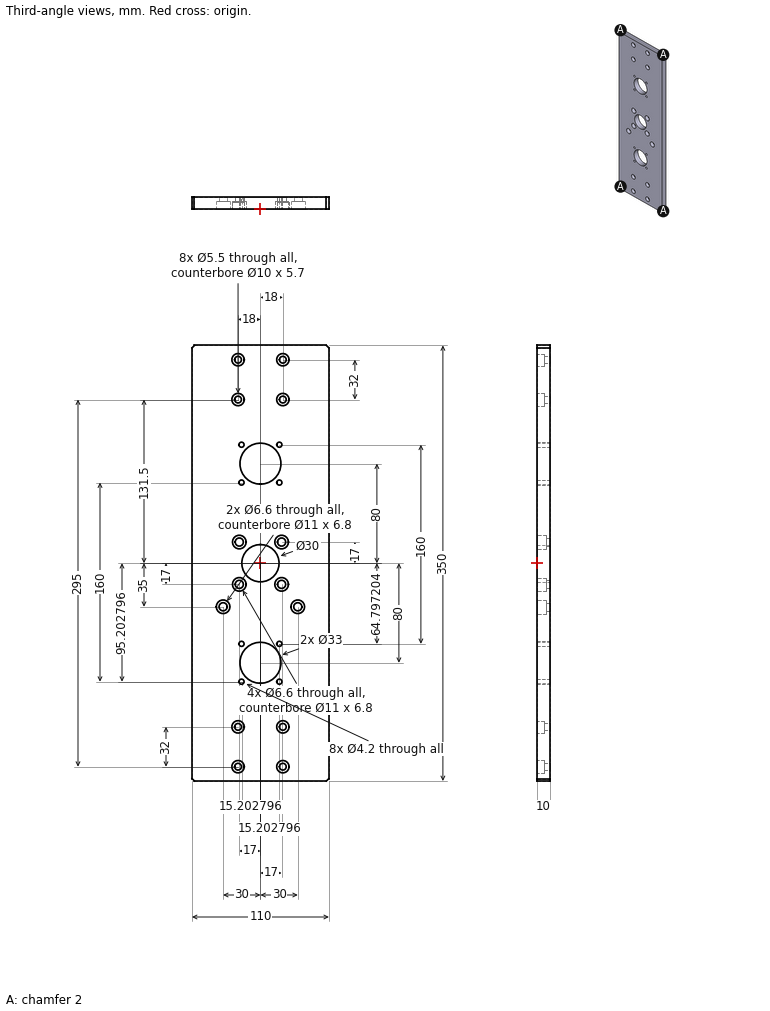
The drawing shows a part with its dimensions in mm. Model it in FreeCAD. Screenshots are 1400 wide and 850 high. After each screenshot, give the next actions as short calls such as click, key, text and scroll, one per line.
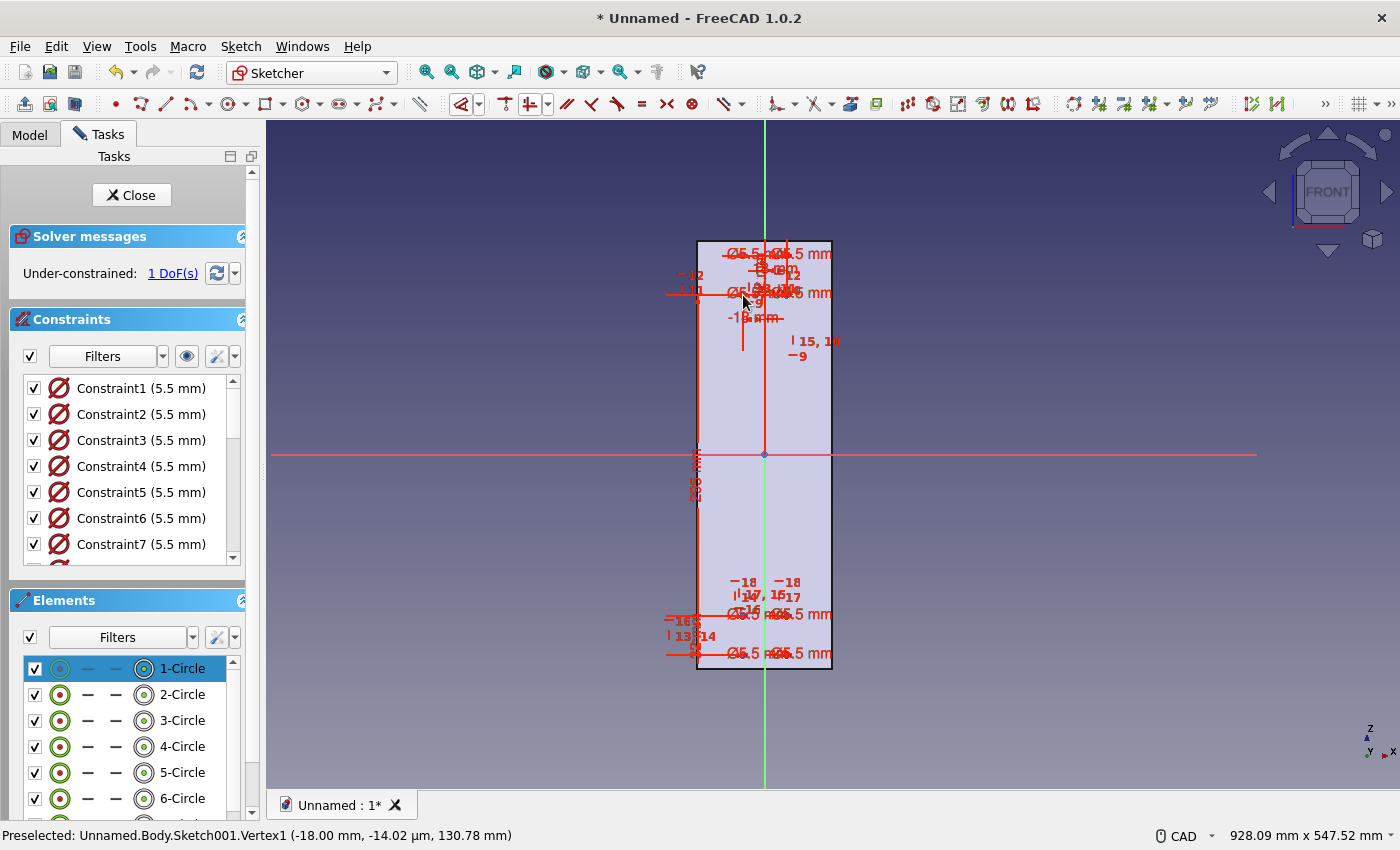
key(i)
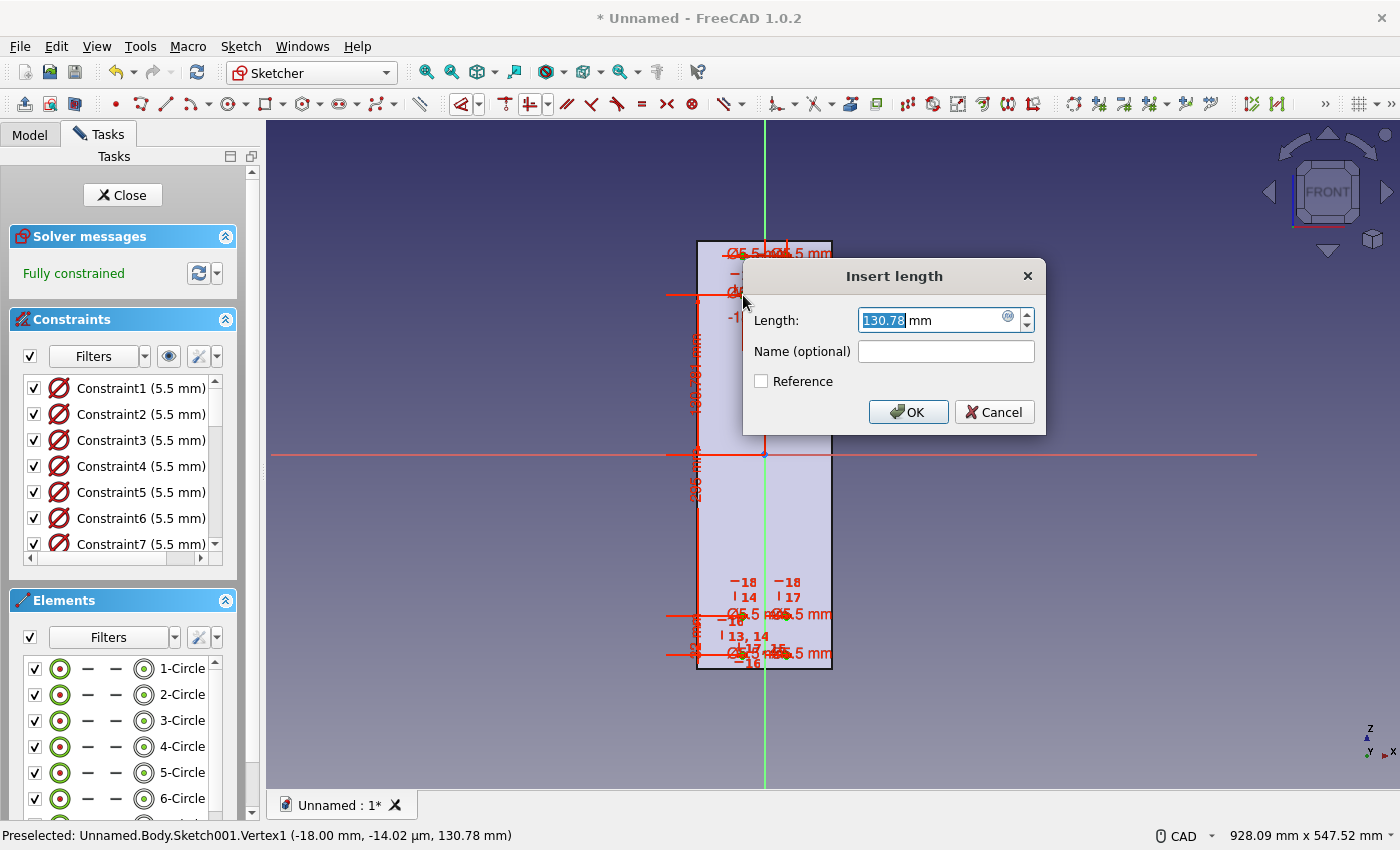
text(131.5)
key(Return)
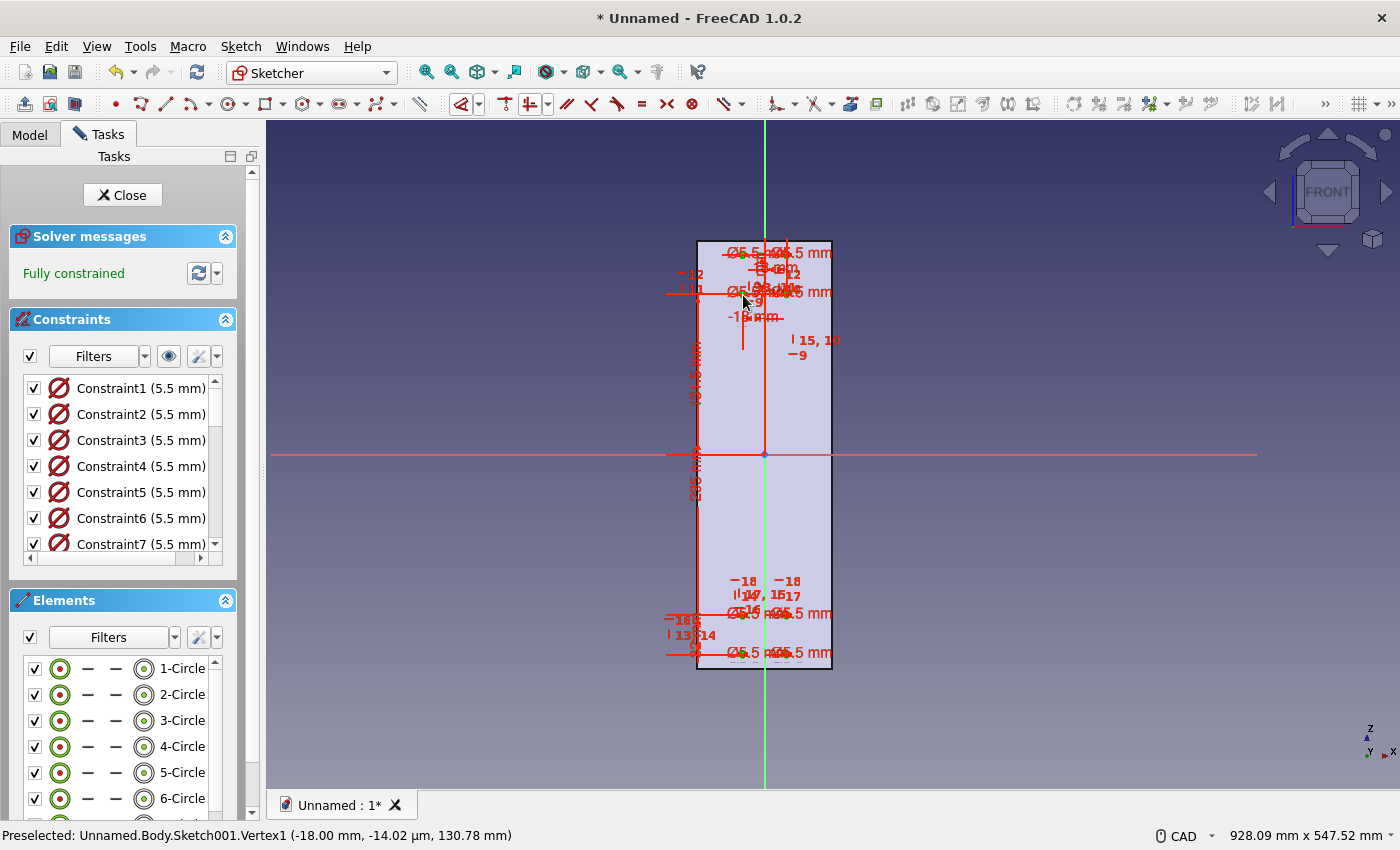
click(123, 195)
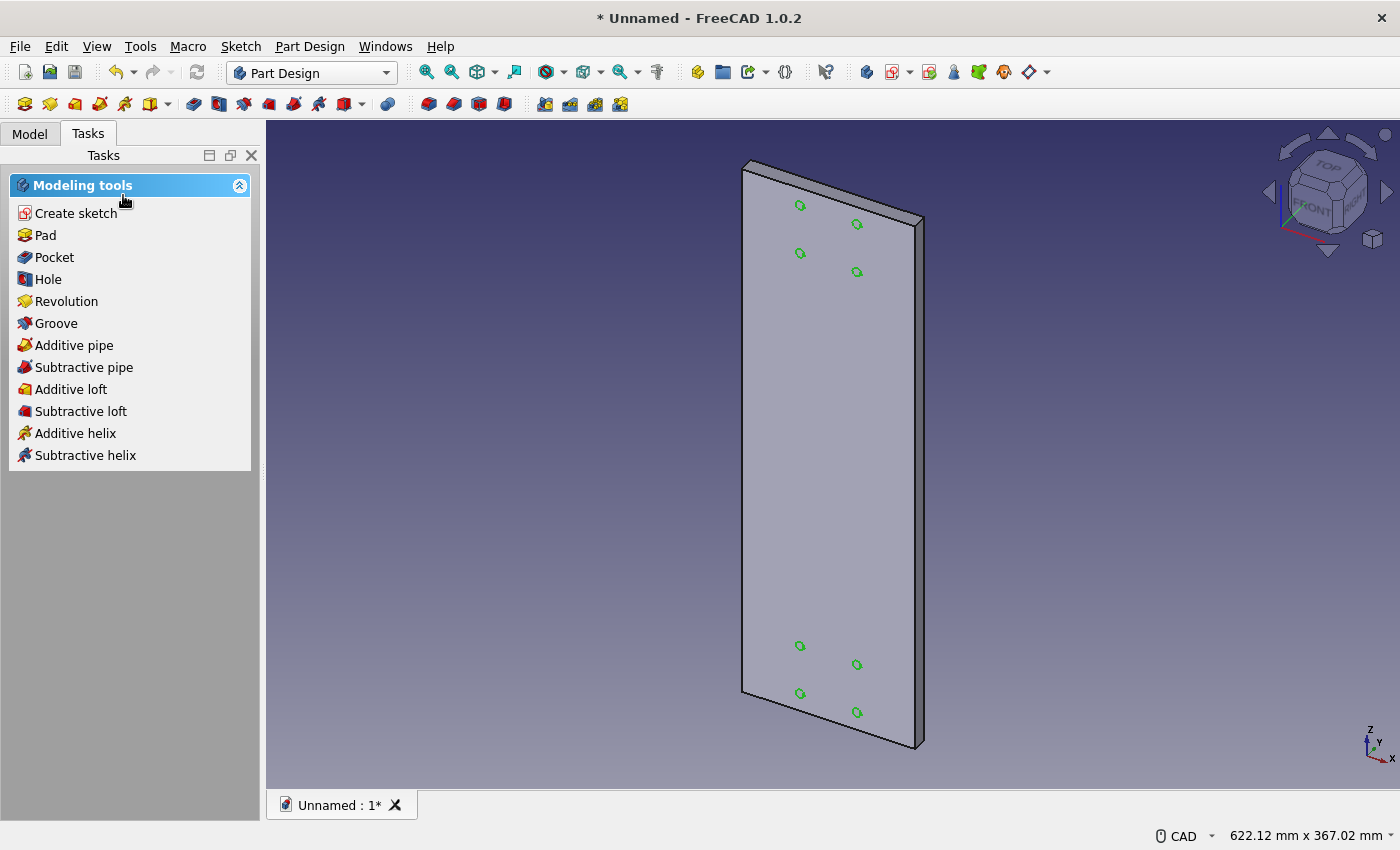
click(219, 104)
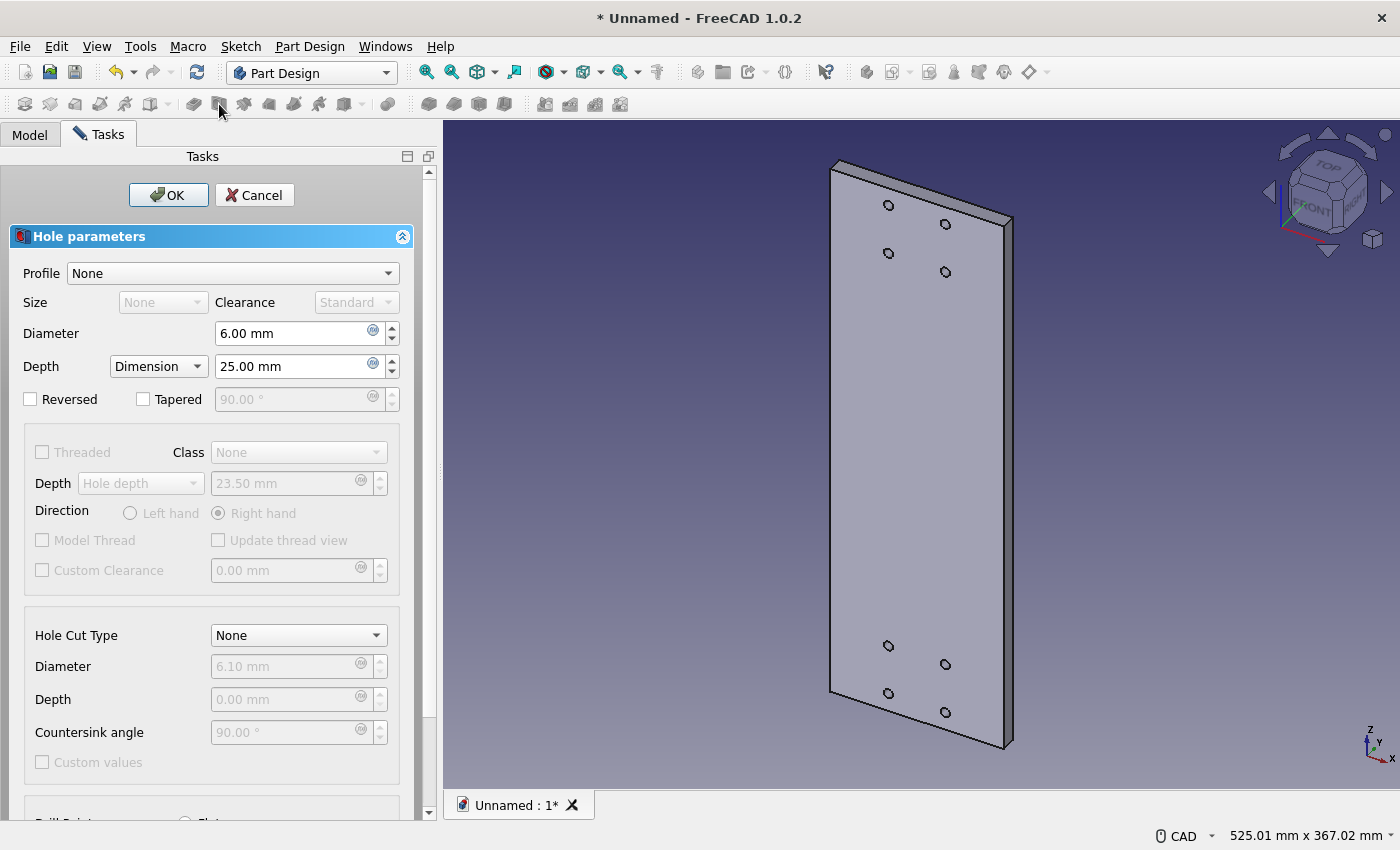
triple_click(300, 334)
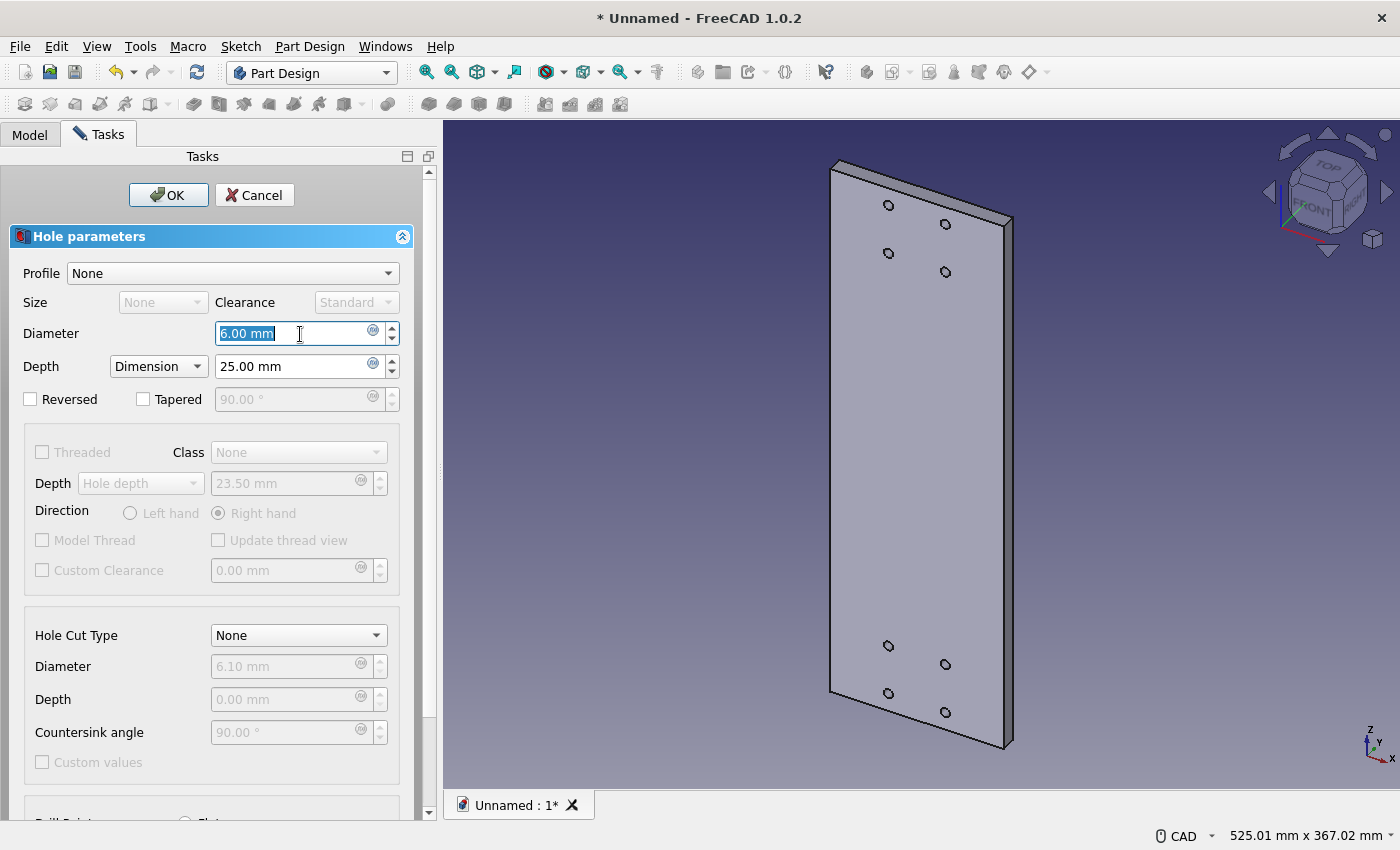
text(5.5)
key(Tab)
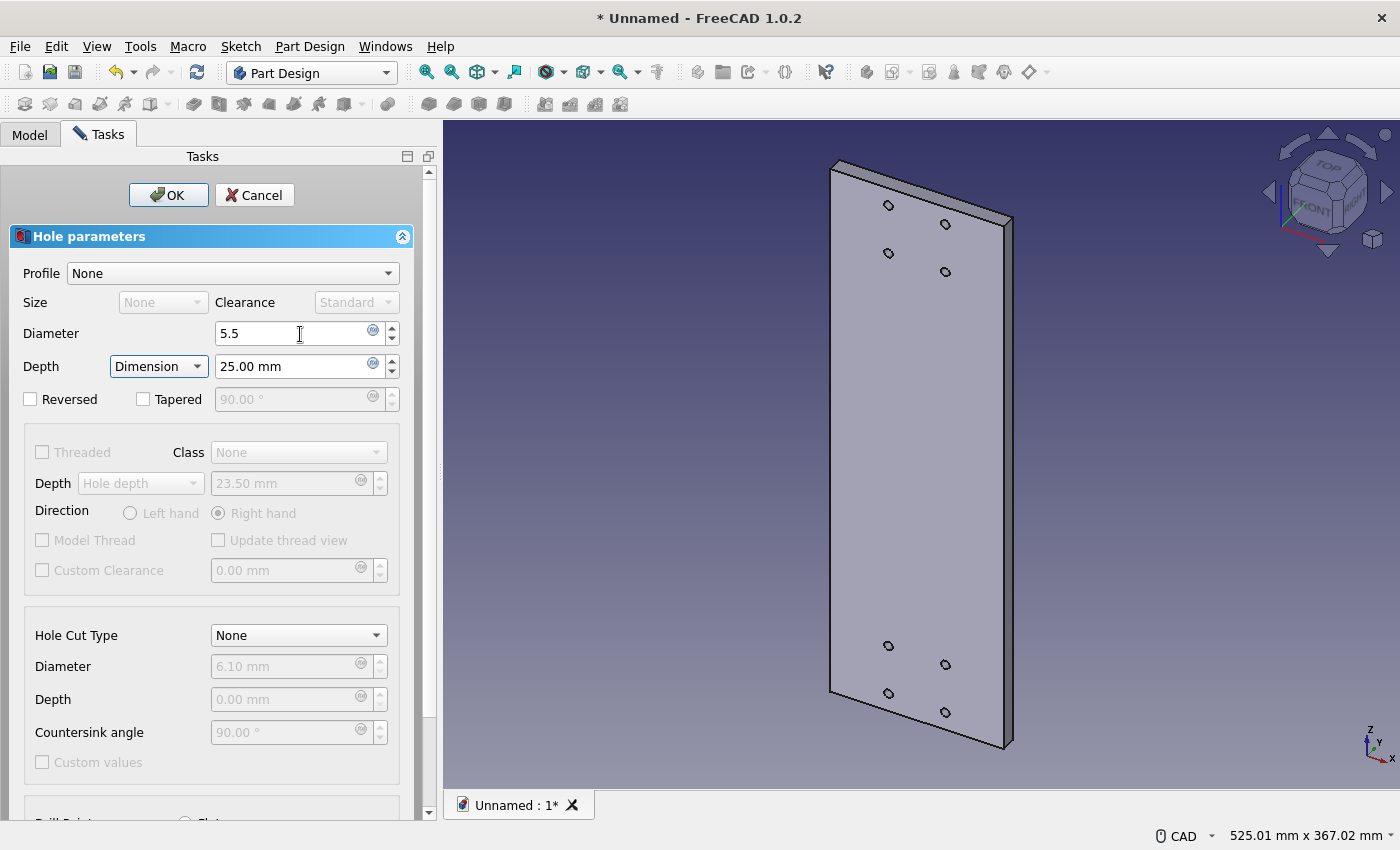
click(160, 366)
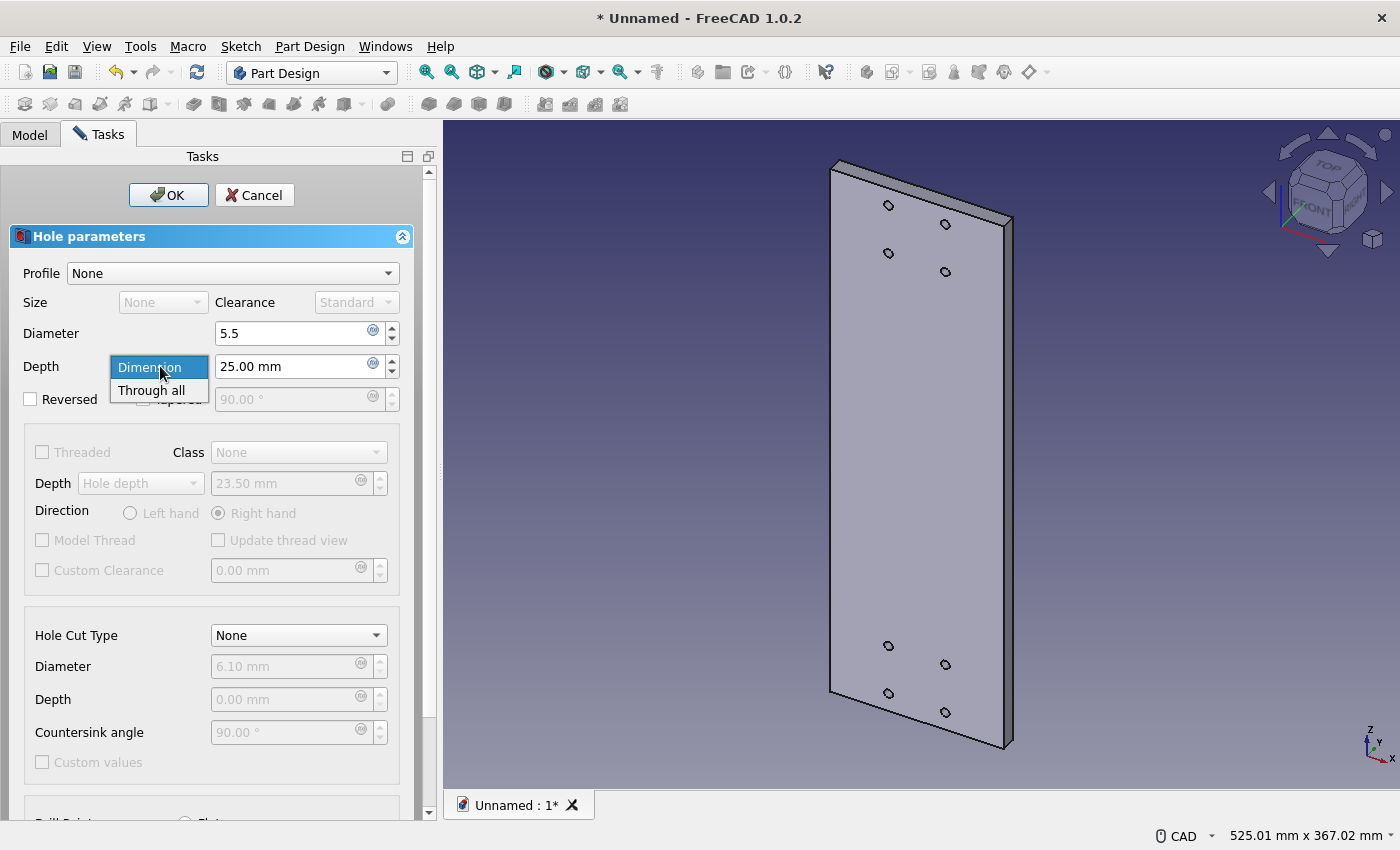
click(158, 390)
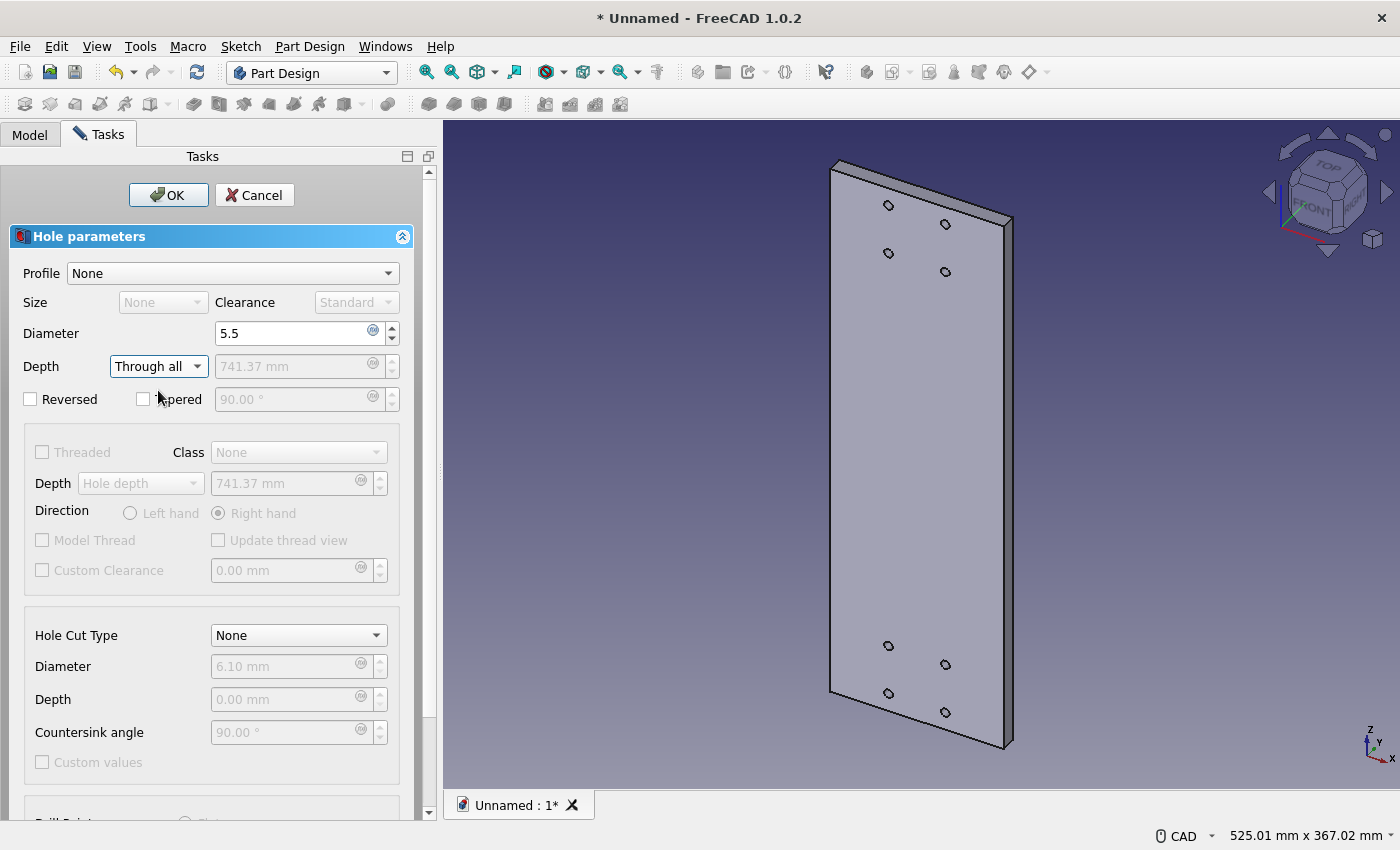
click(300, 636)